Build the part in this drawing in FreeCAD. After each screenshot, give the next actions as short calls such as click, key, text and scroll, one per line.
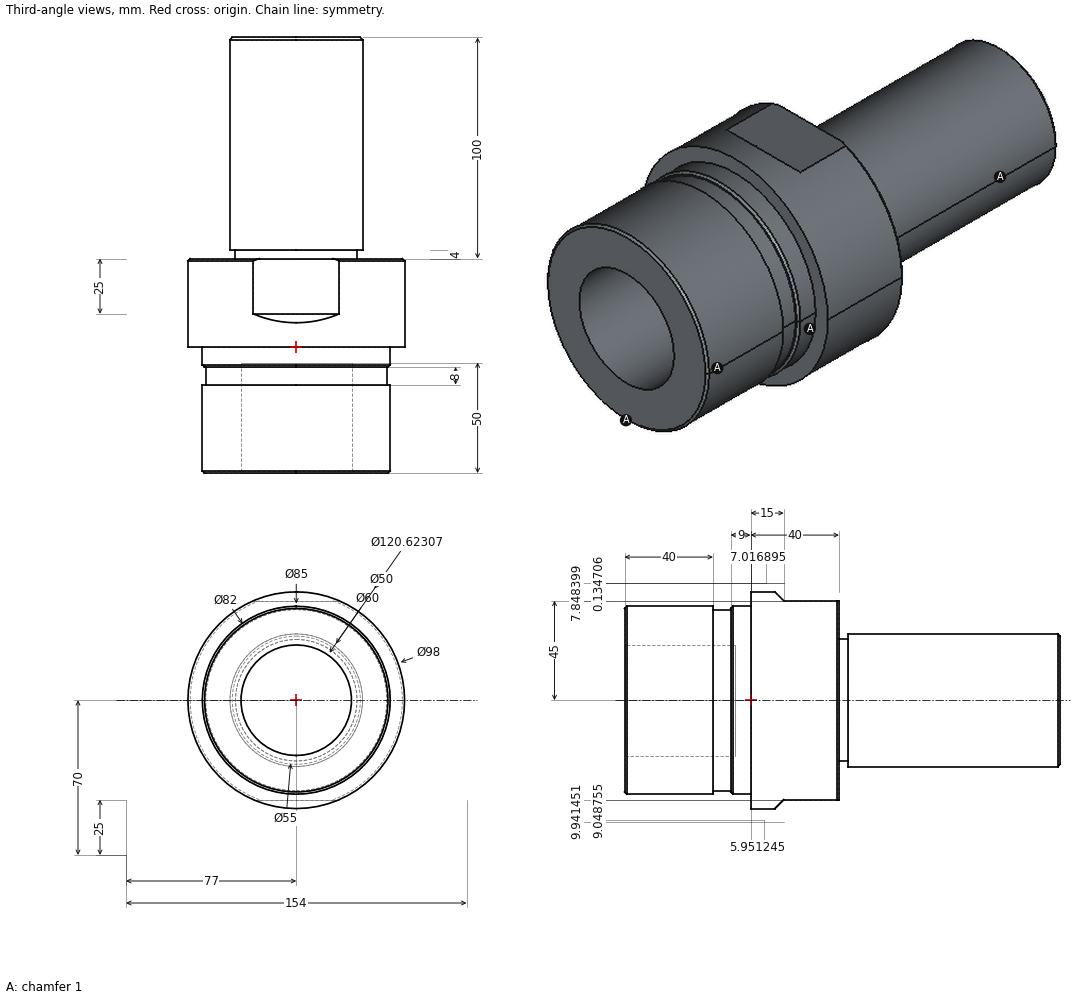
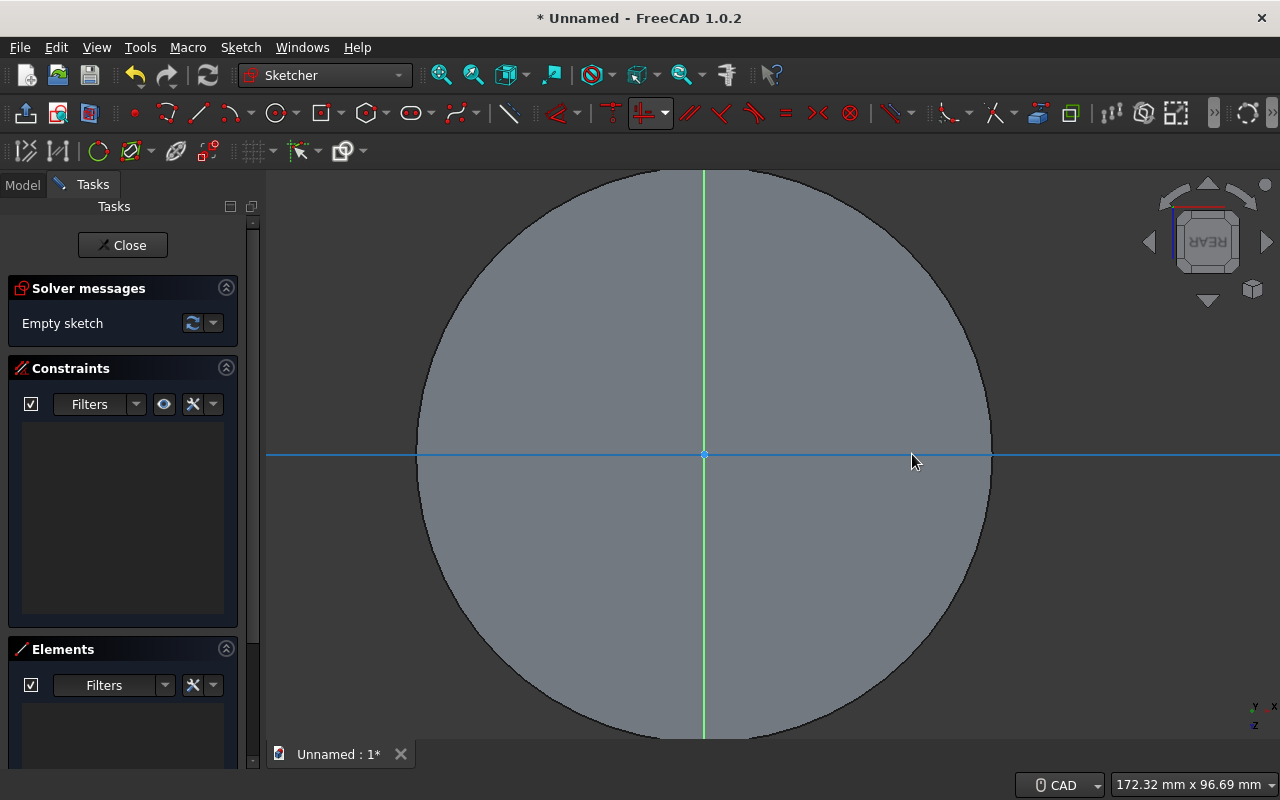
click(276, 114)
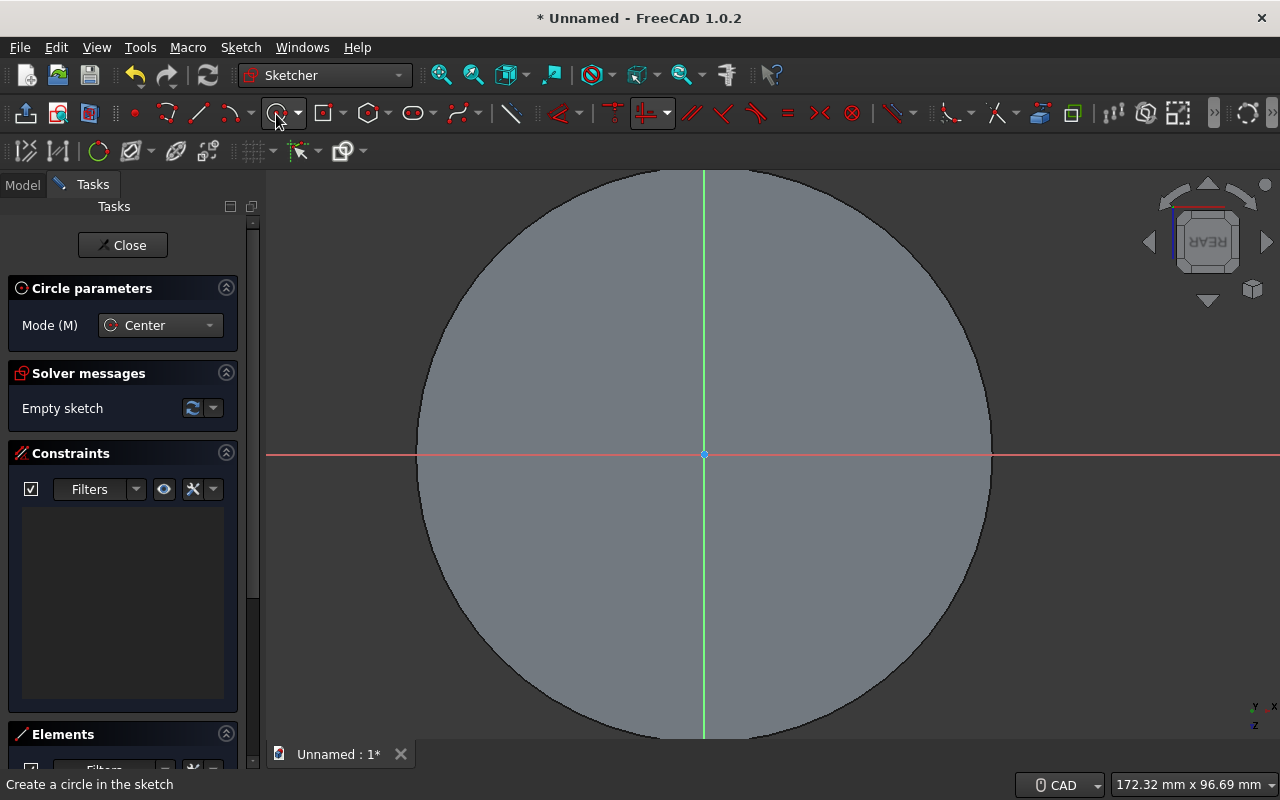
click(704, 454)
click(829, 330)
key(Escape)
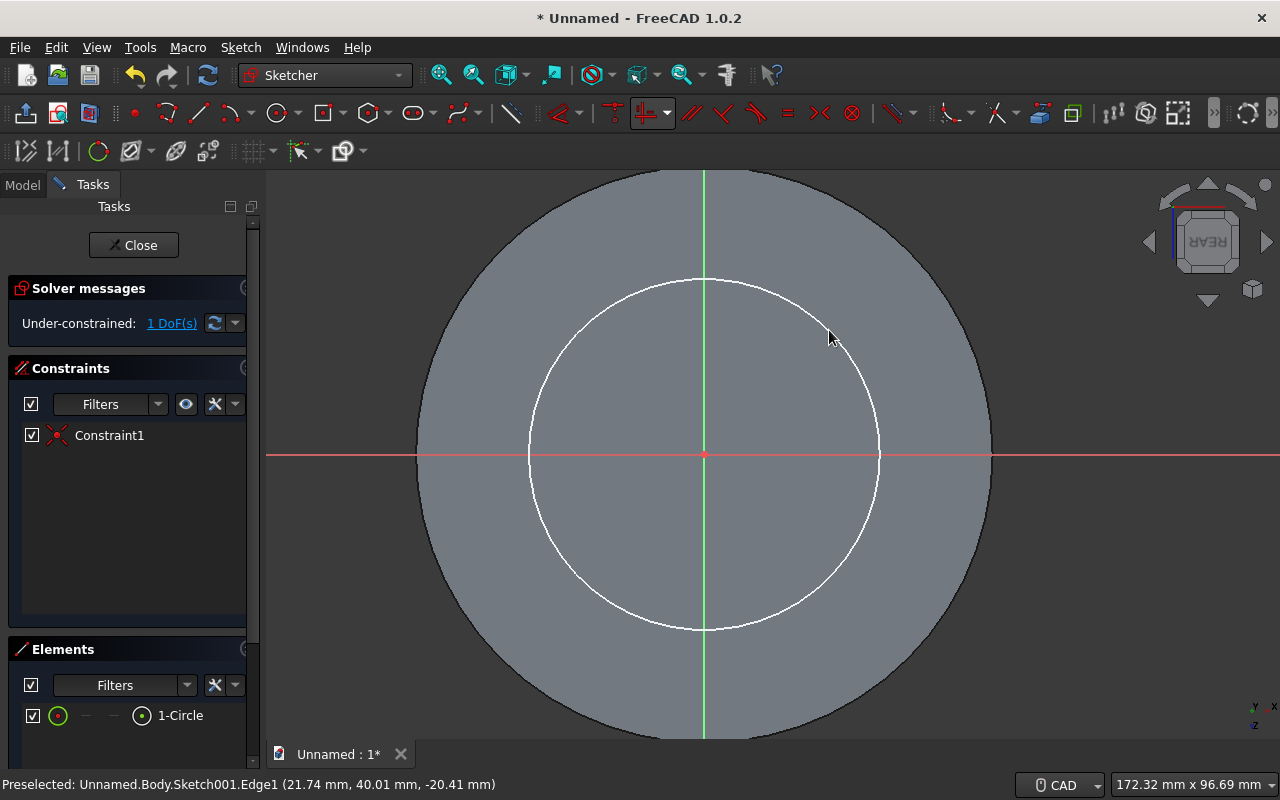
click(558, 114)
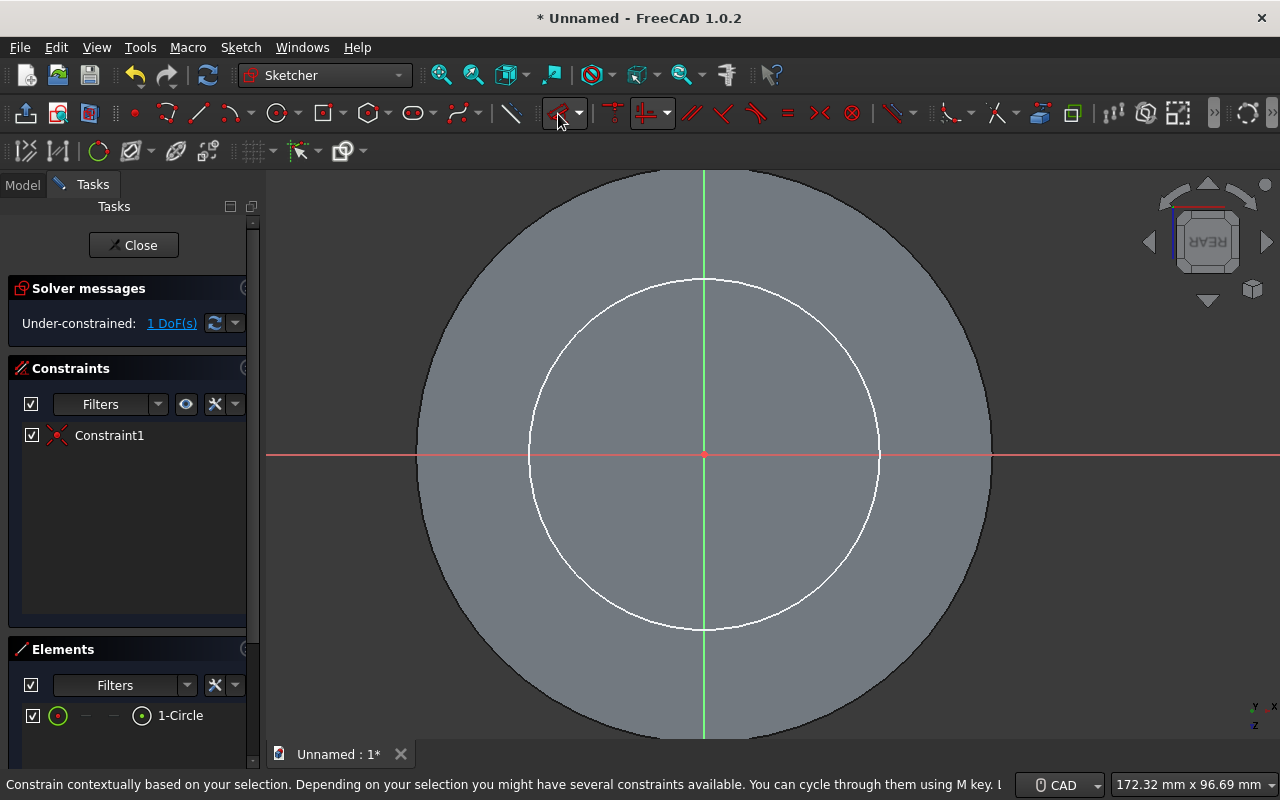
click(828, 330)
click(851, 307)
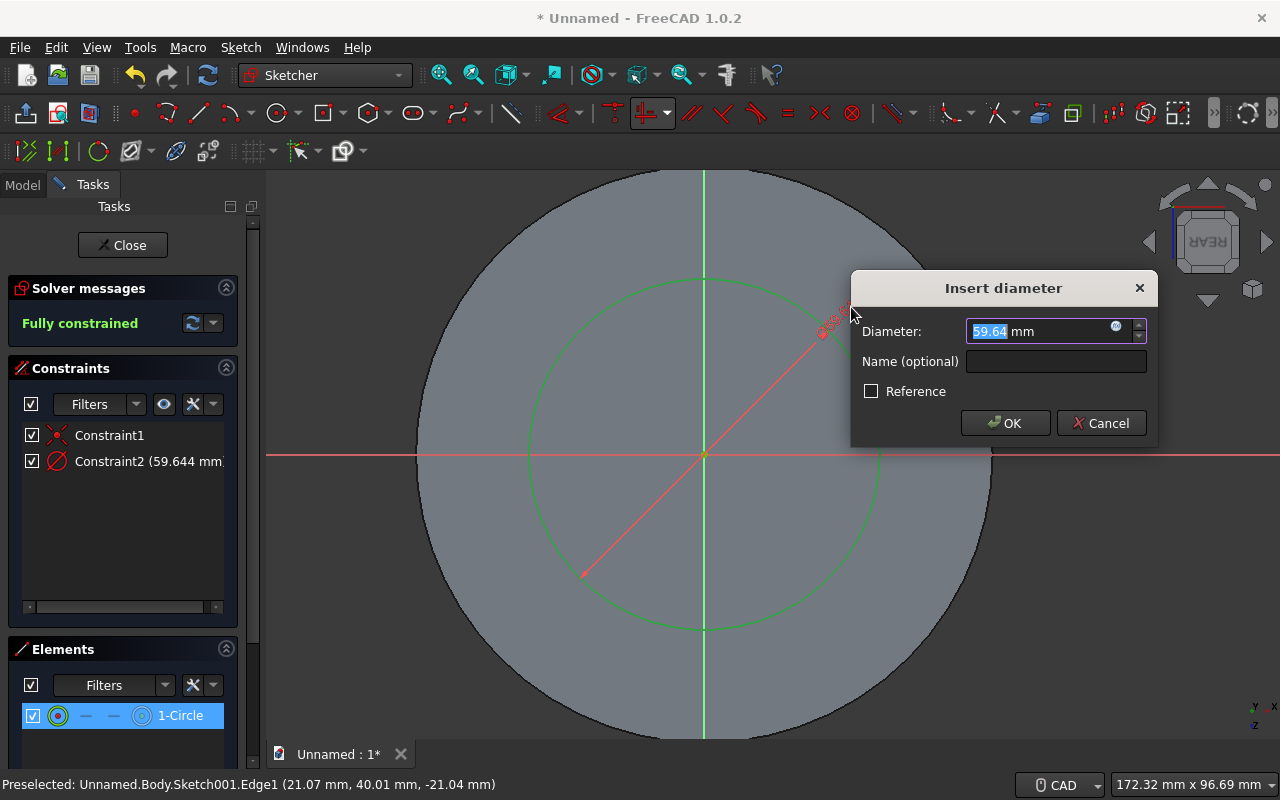
text(60)
key(Return)
key(Escape)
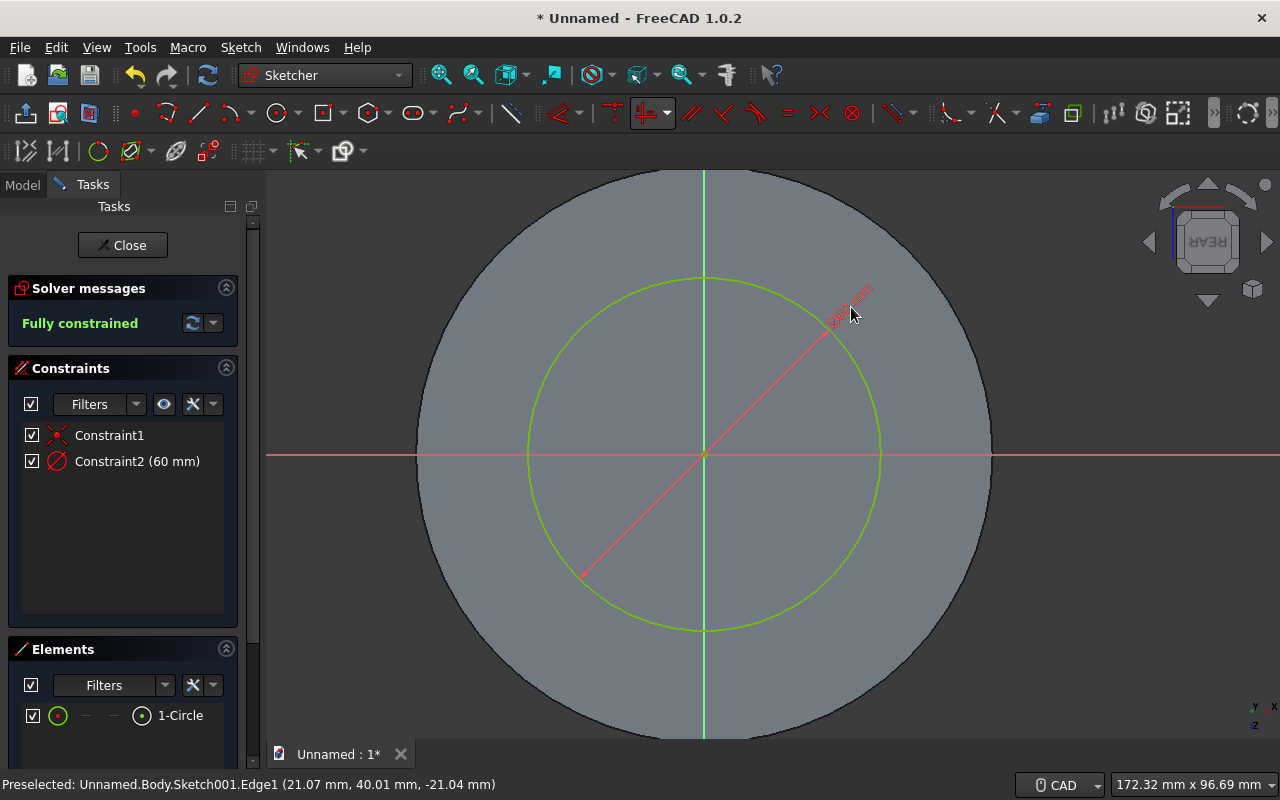
click(123, 245)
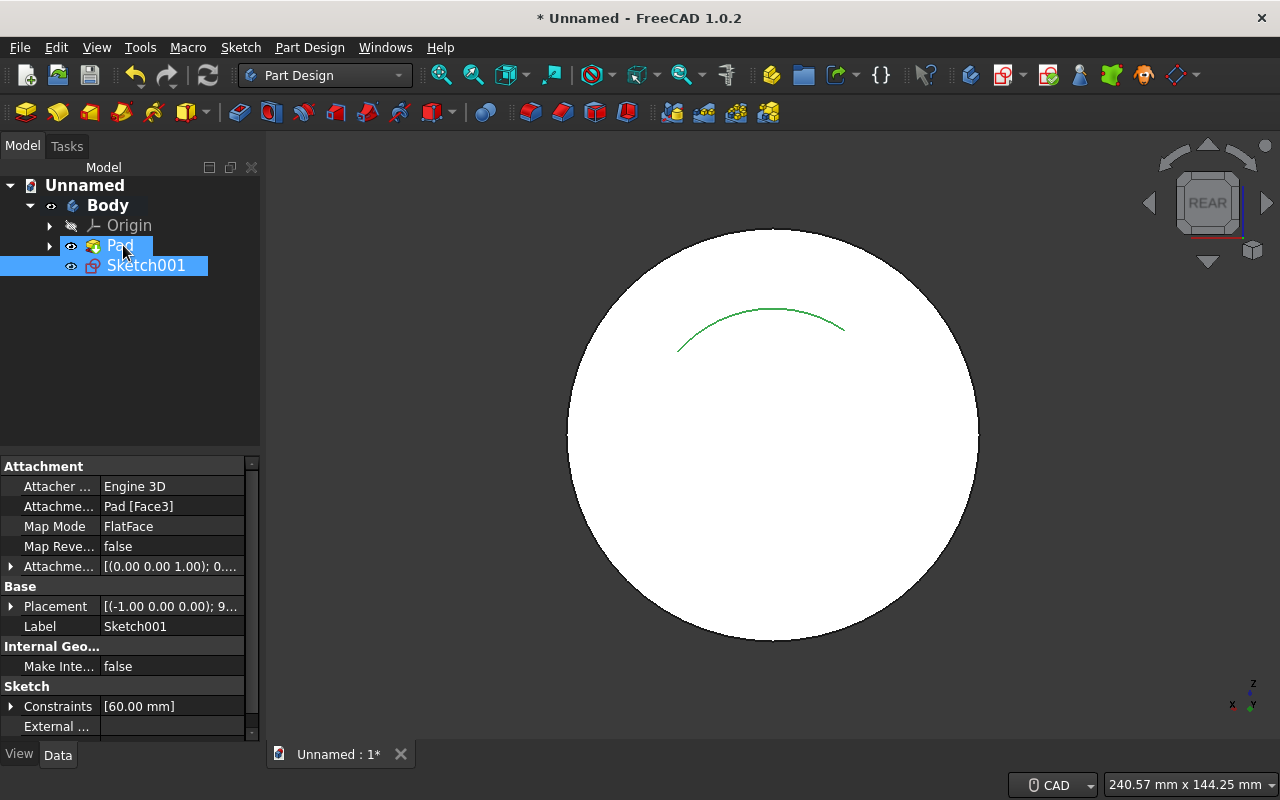
click(26, 112)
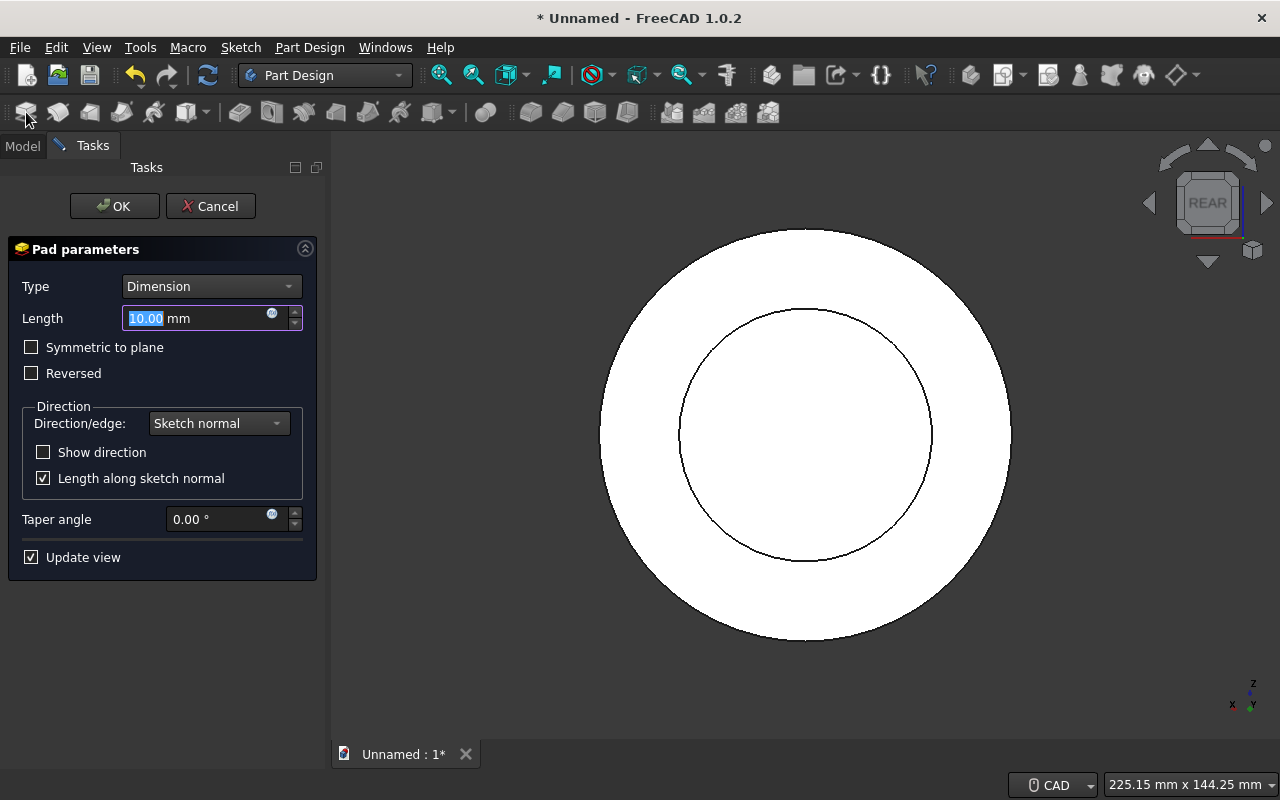
text(100)
key(Tab)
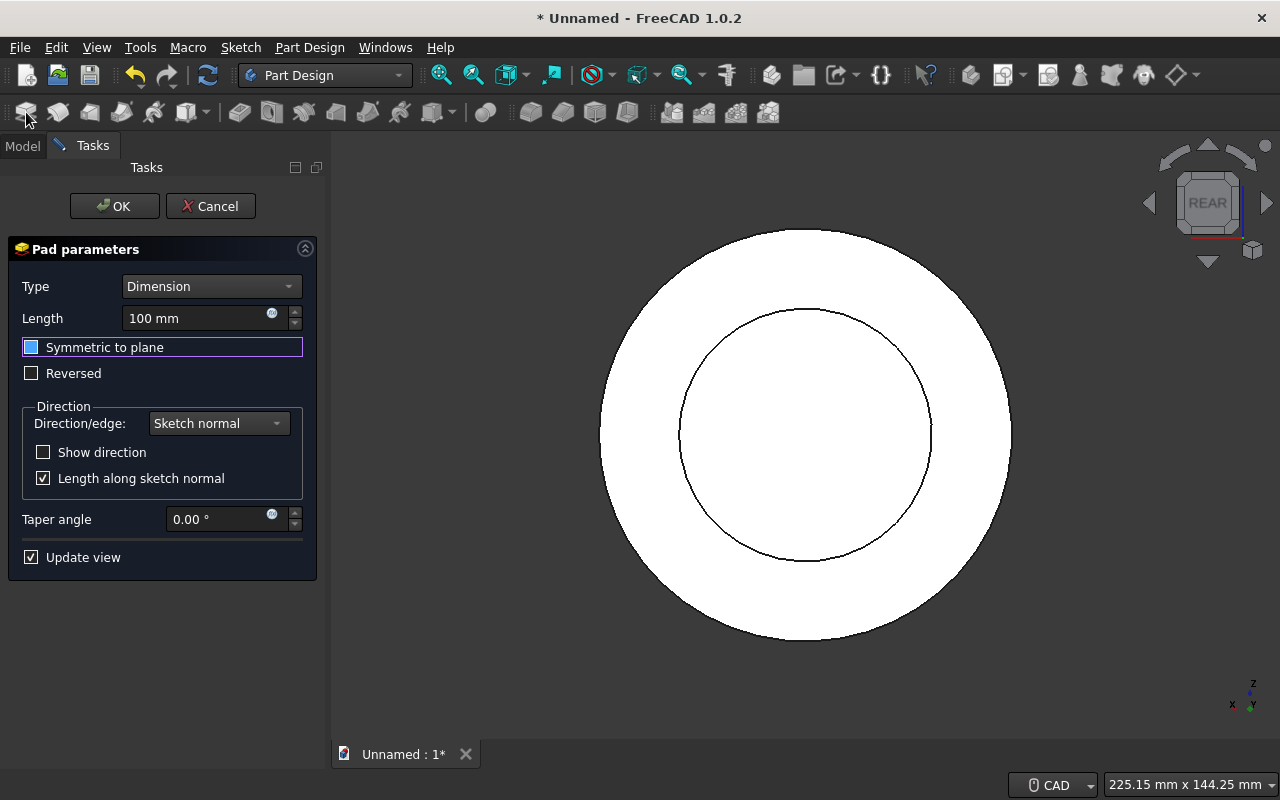
click(115, 206)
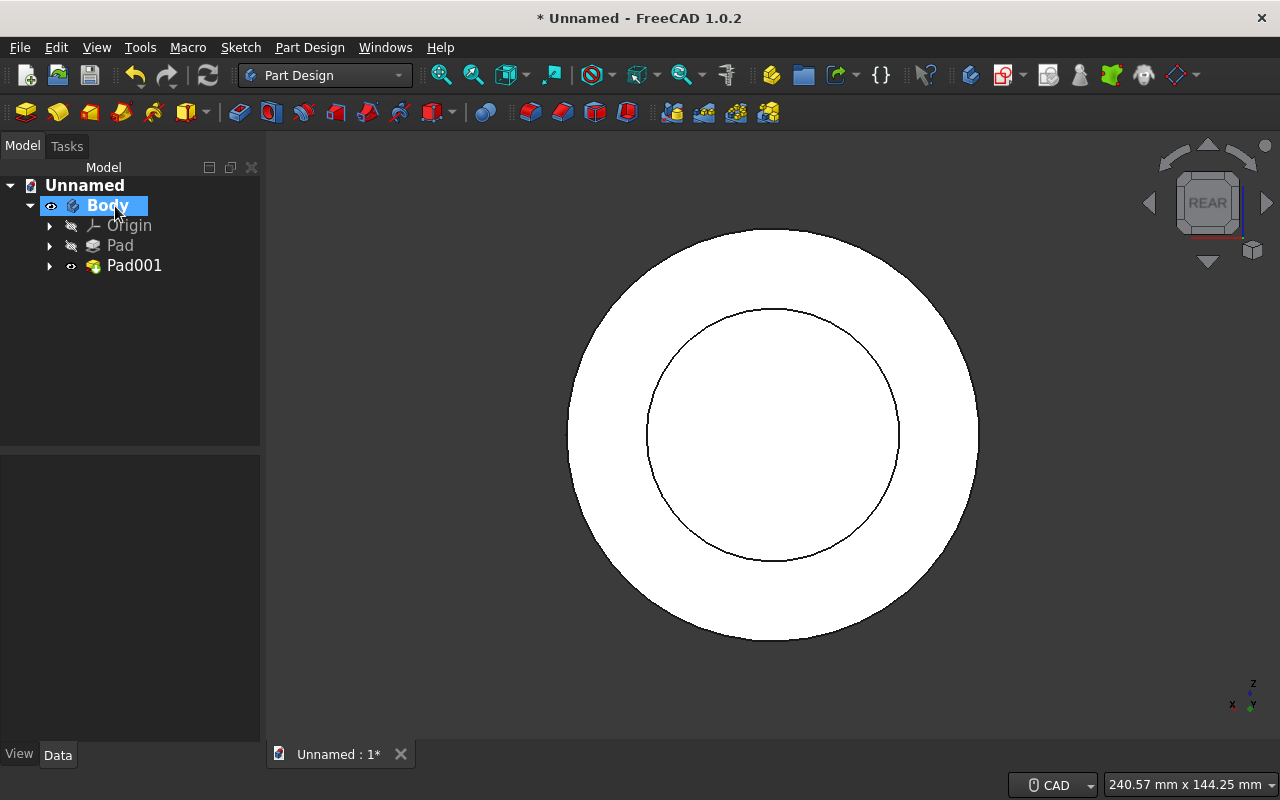
click(1004, 76)